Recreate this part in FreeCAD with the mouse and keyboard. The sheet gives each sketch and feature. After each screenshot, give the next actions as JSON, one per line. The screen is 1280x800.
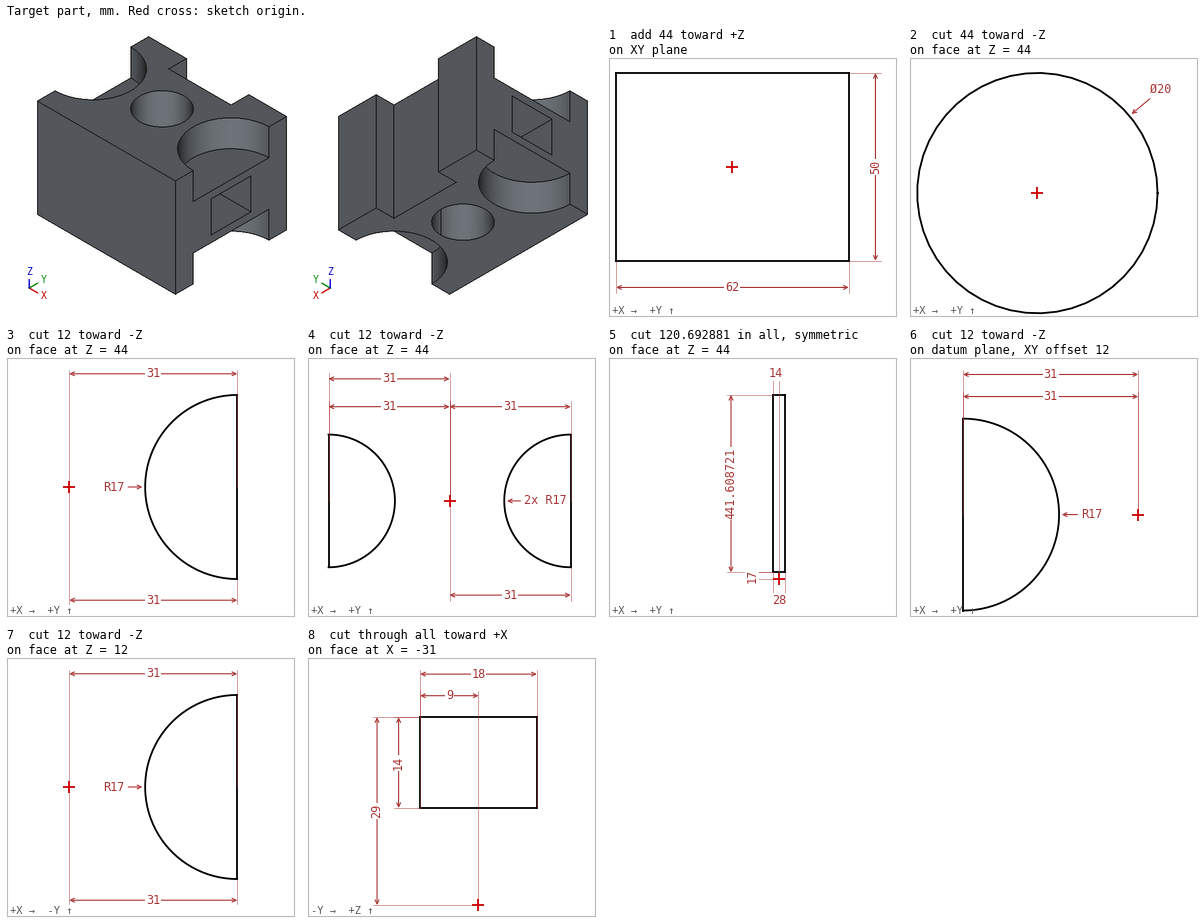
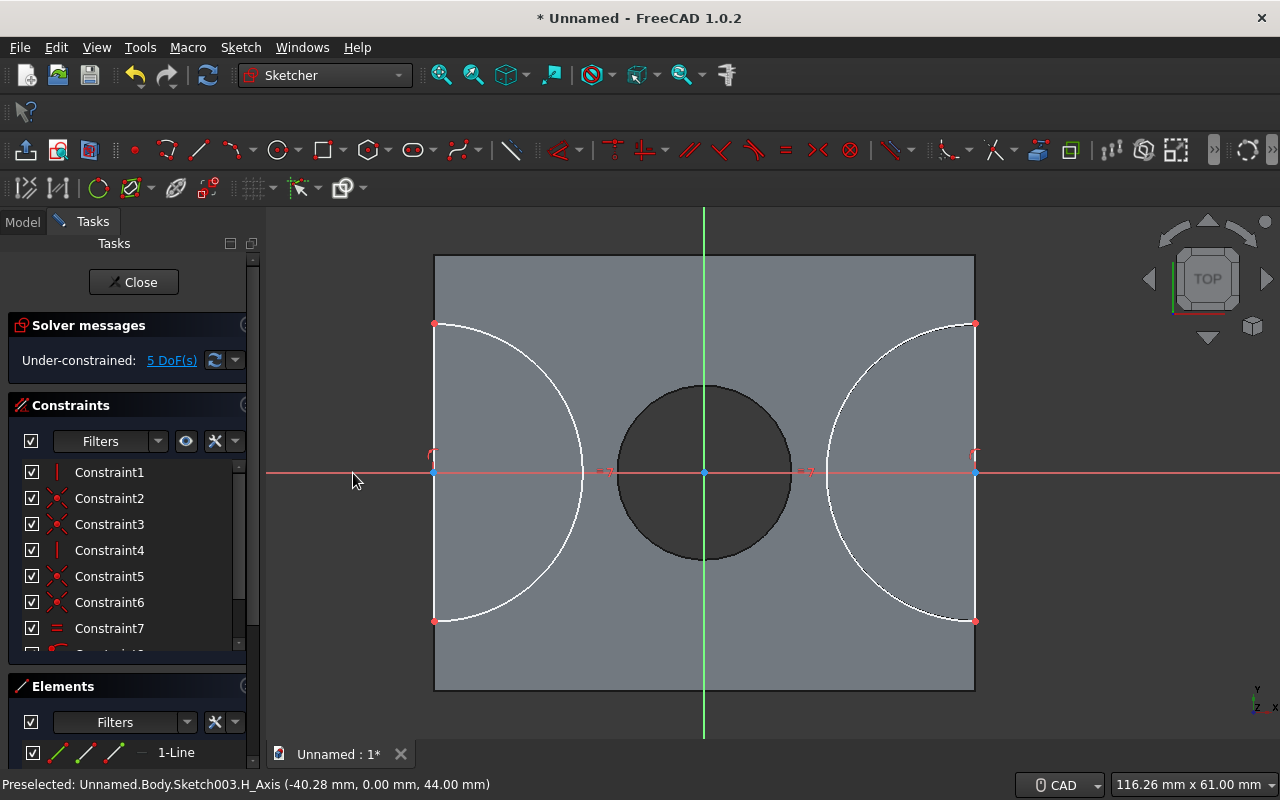
{"action": "left_click", "coordinate": [558, 150]}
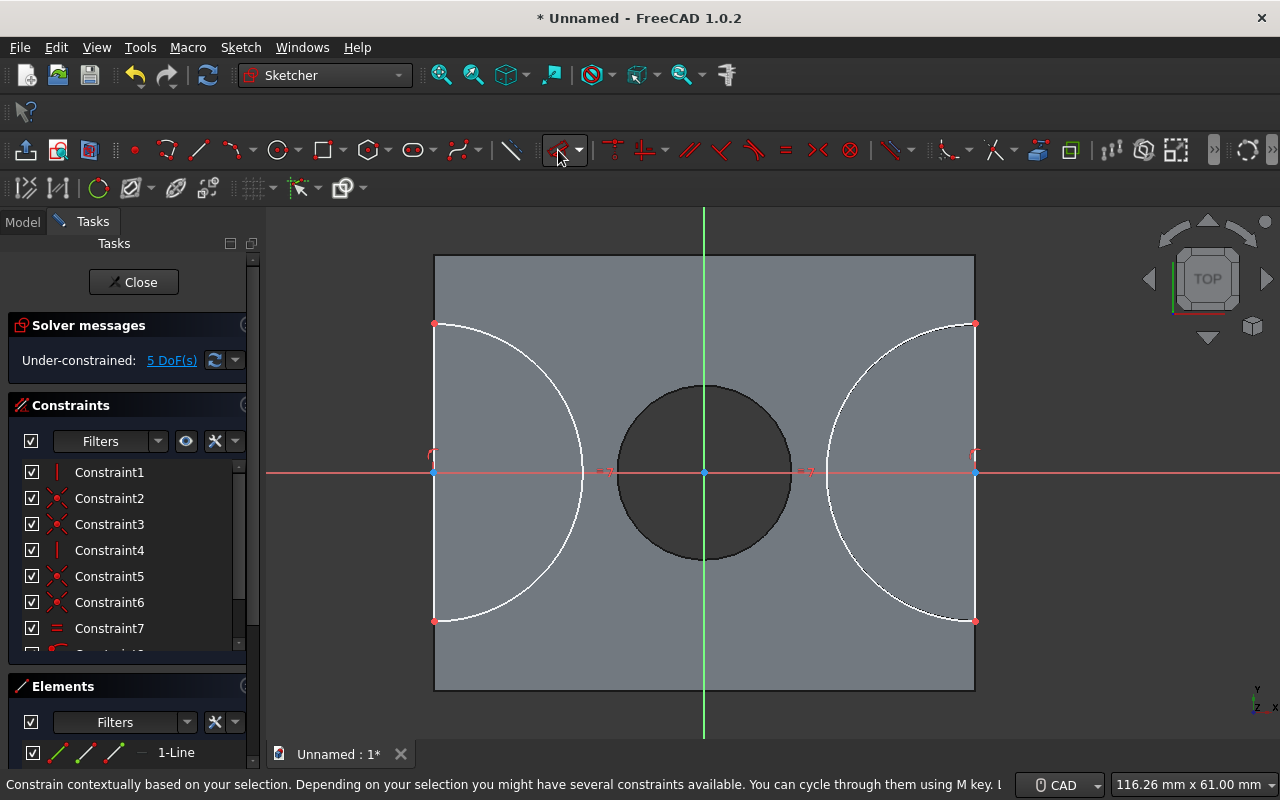
{"action": "left_click", "coordinate": [855, 385]}
{"action": "left_click", "coordinate": [829, 366]}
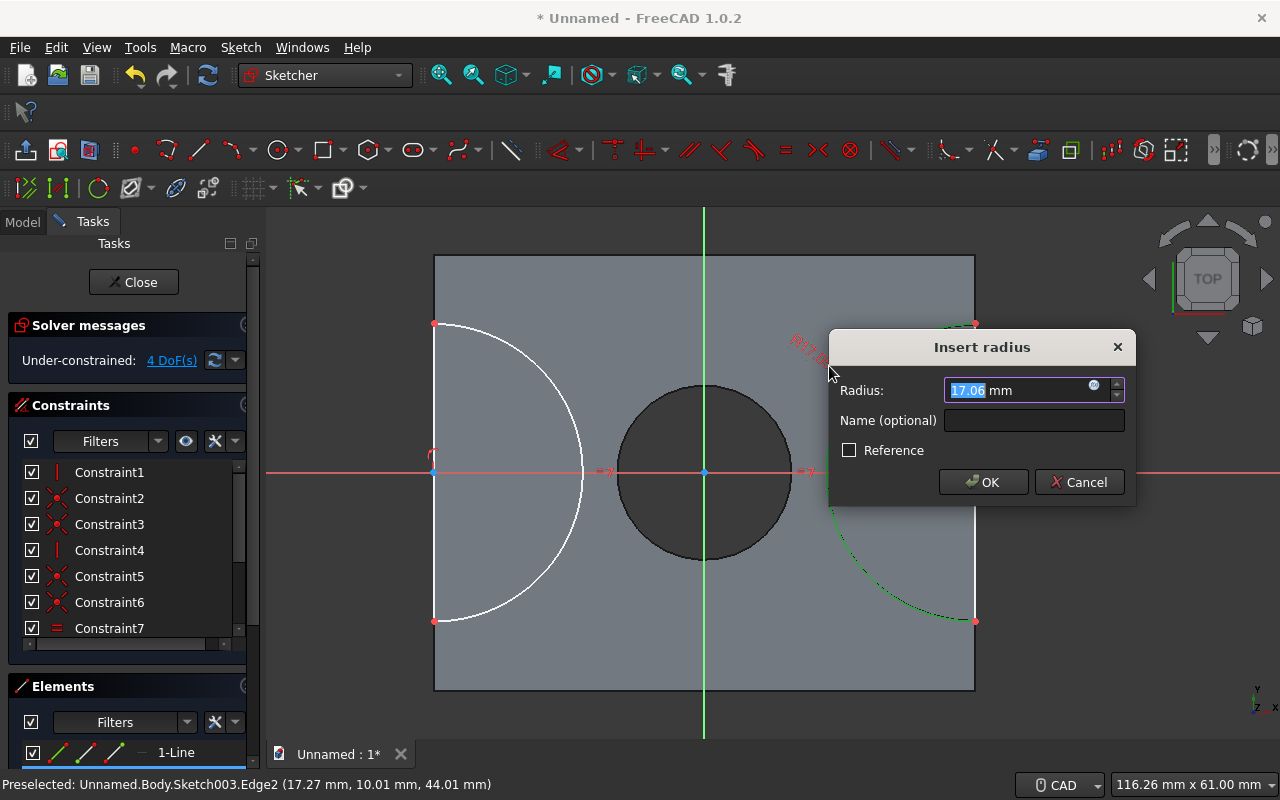
{"action": "type", "text": "17"}
{"action": "key", "text": "Return"}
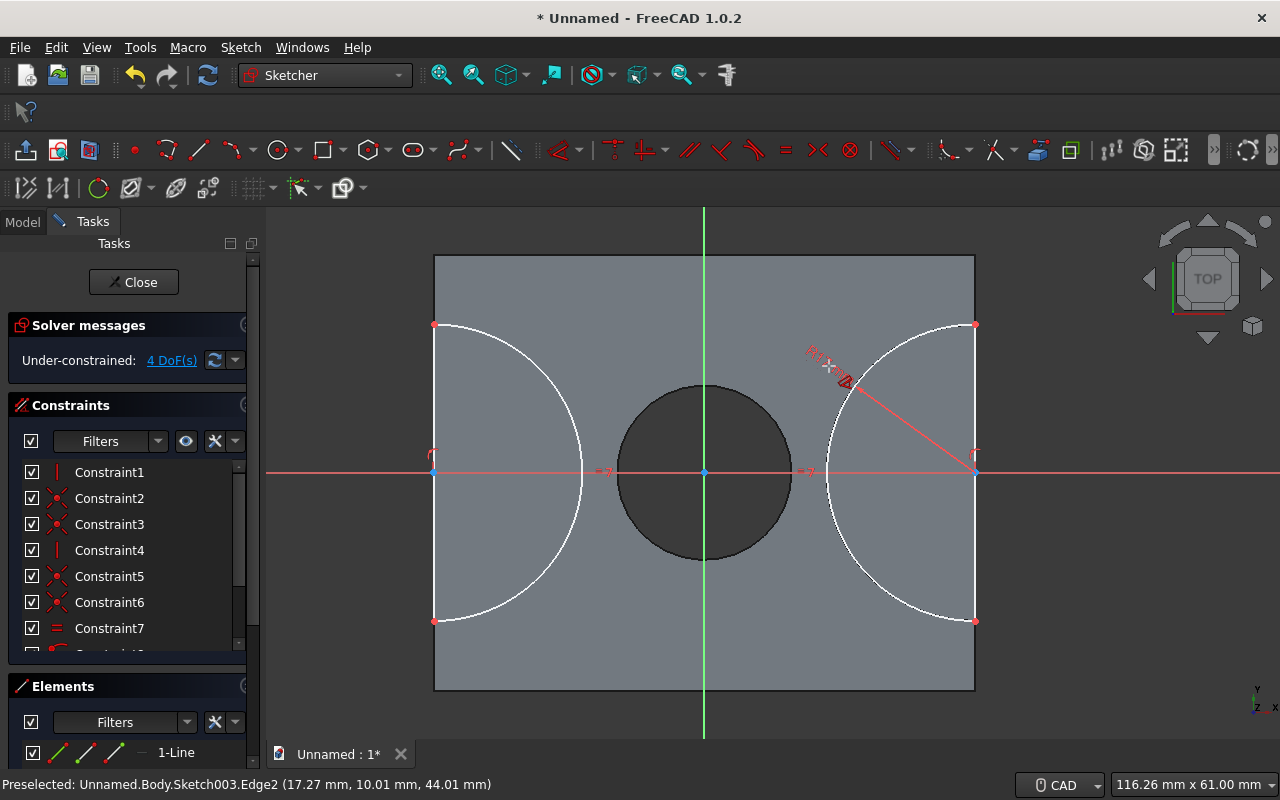
{"action": "left_click", "coordinate": [975, 621]}
{"action": "left_click", "coordinate": [840, 655]}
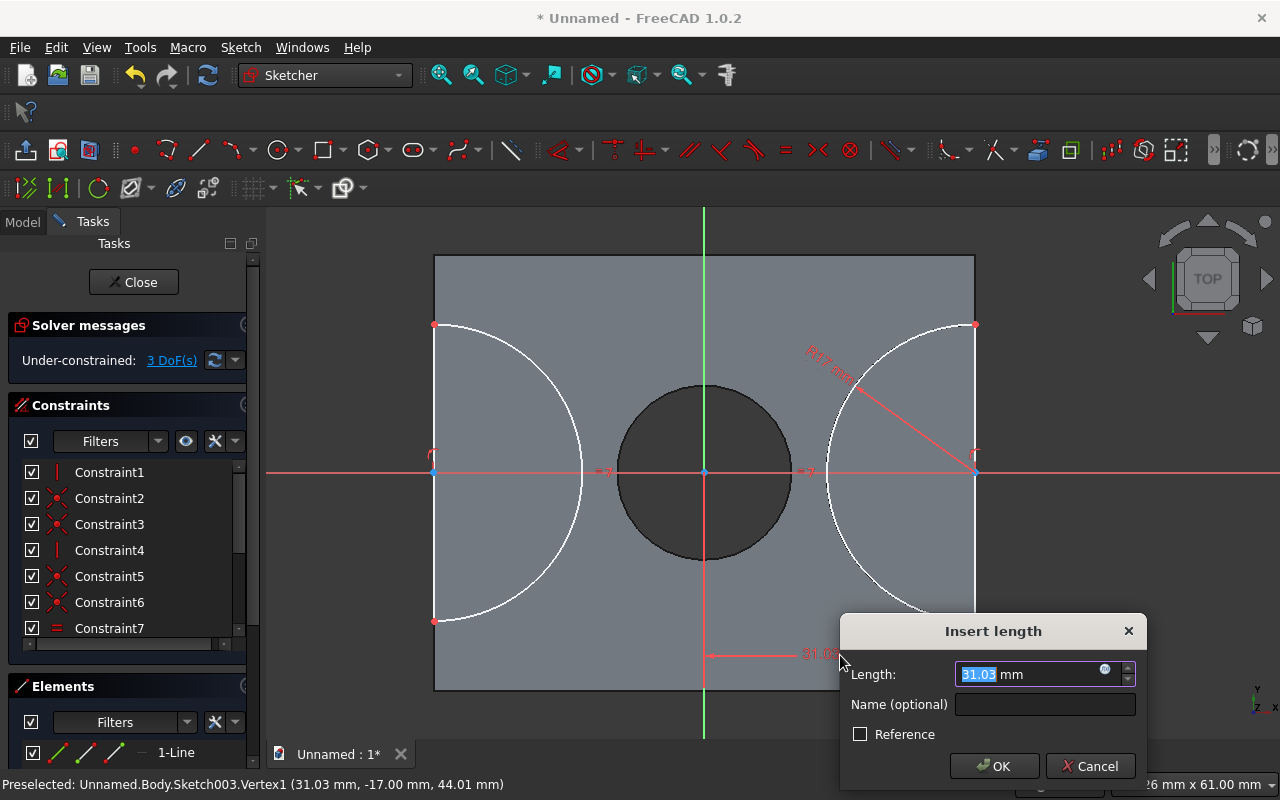
{"action": "type", "text": "31"}
{"action": "key", "text": "Return"}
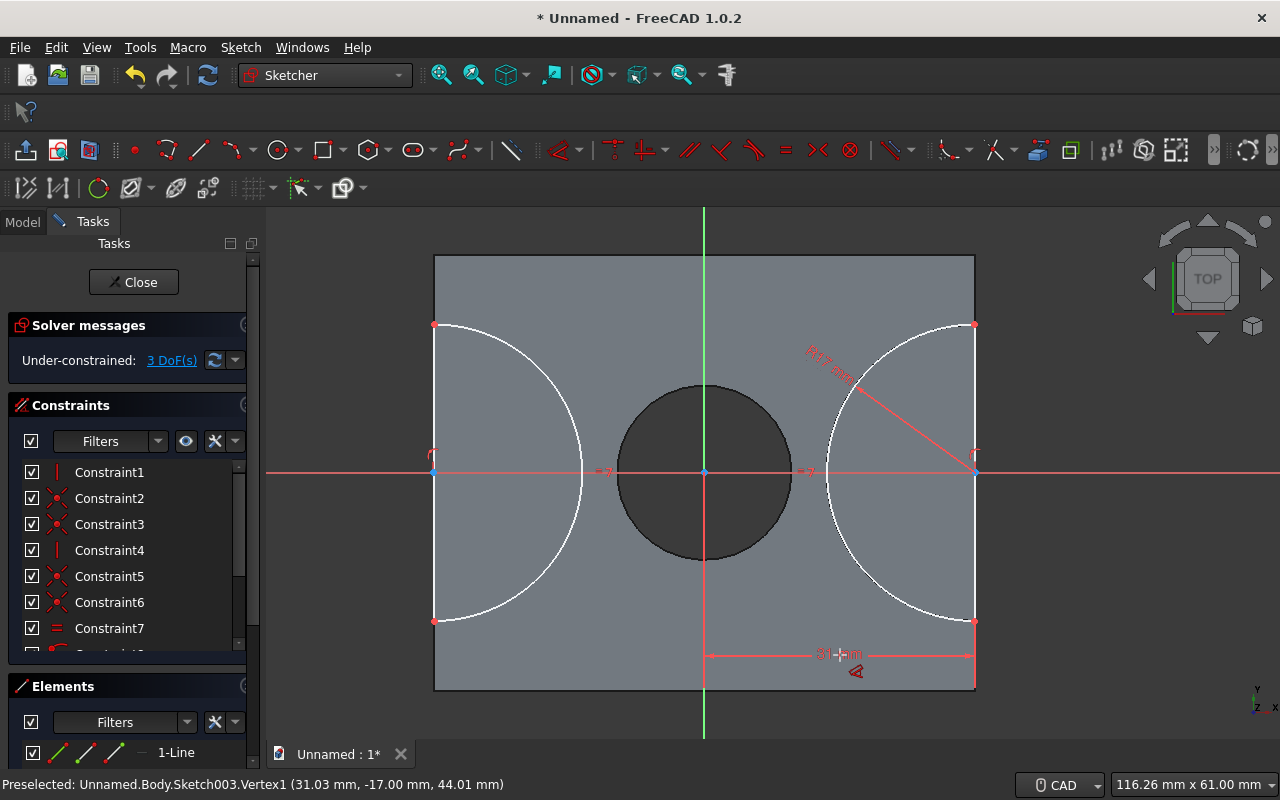
{"action": "left_click", "coordinate": [434, 324]}
{"action": "left_click", "coordinate": [569, 290]}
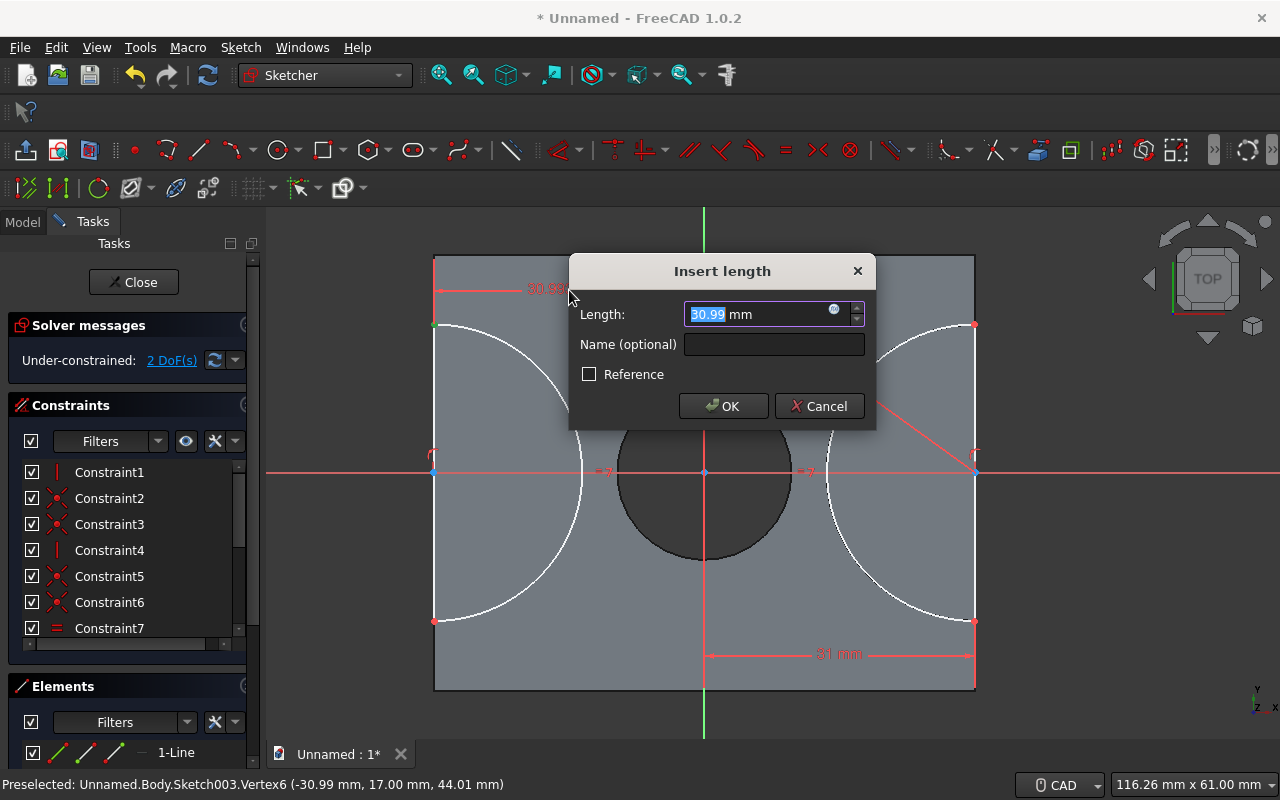
{"action": "type", "text": "31"}
{"action": "key", "text": "Return"}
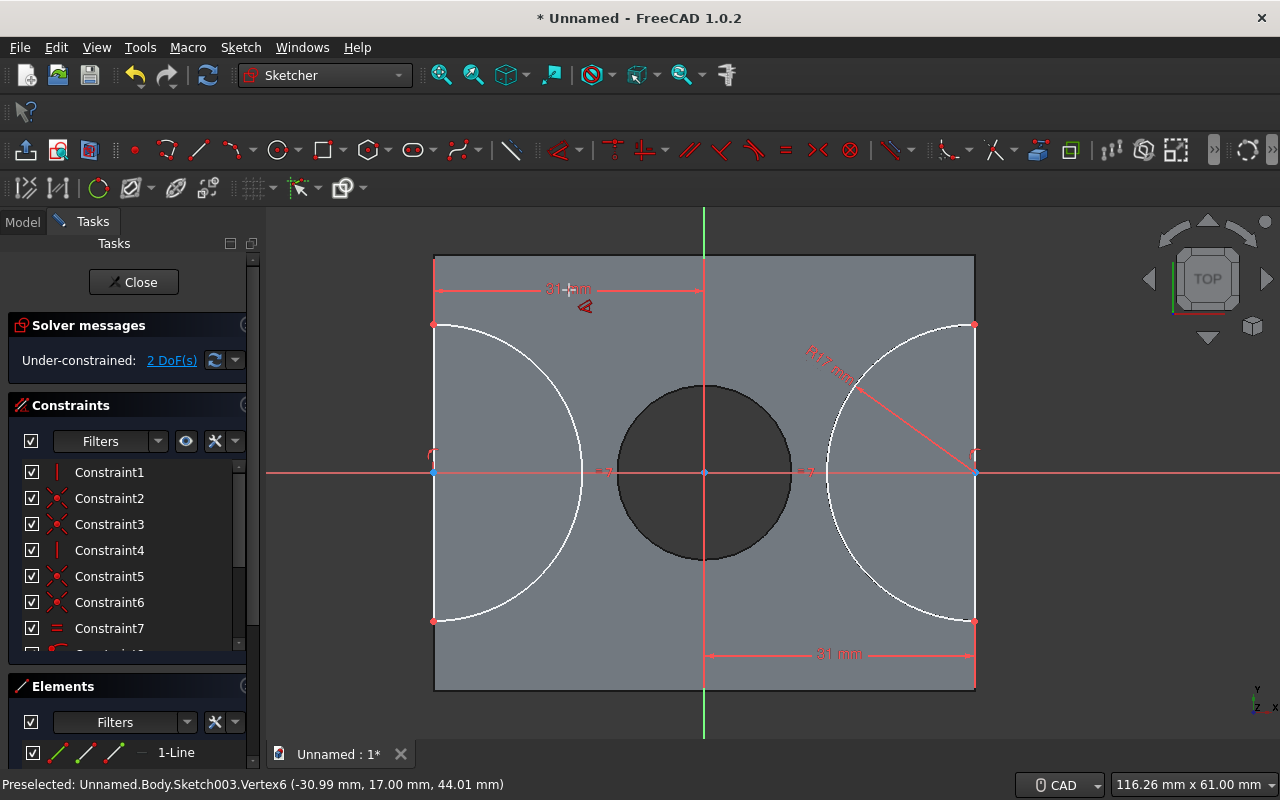
{"action": "left_click", "coordinate": [975, 473]}
{"action": "left_click", "coordinate": [778, 507]}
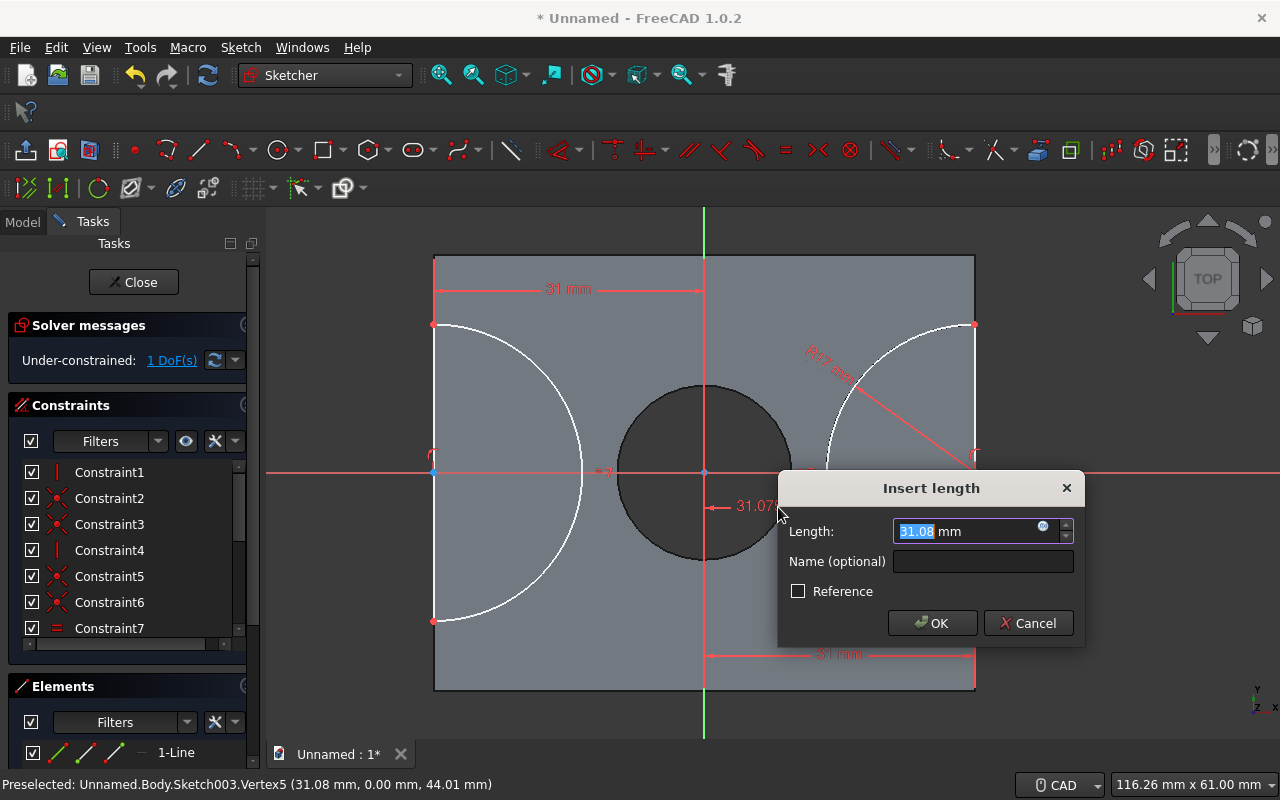
{"action": "type", "text": "31"}
{"action": "key", "text": "Return"}